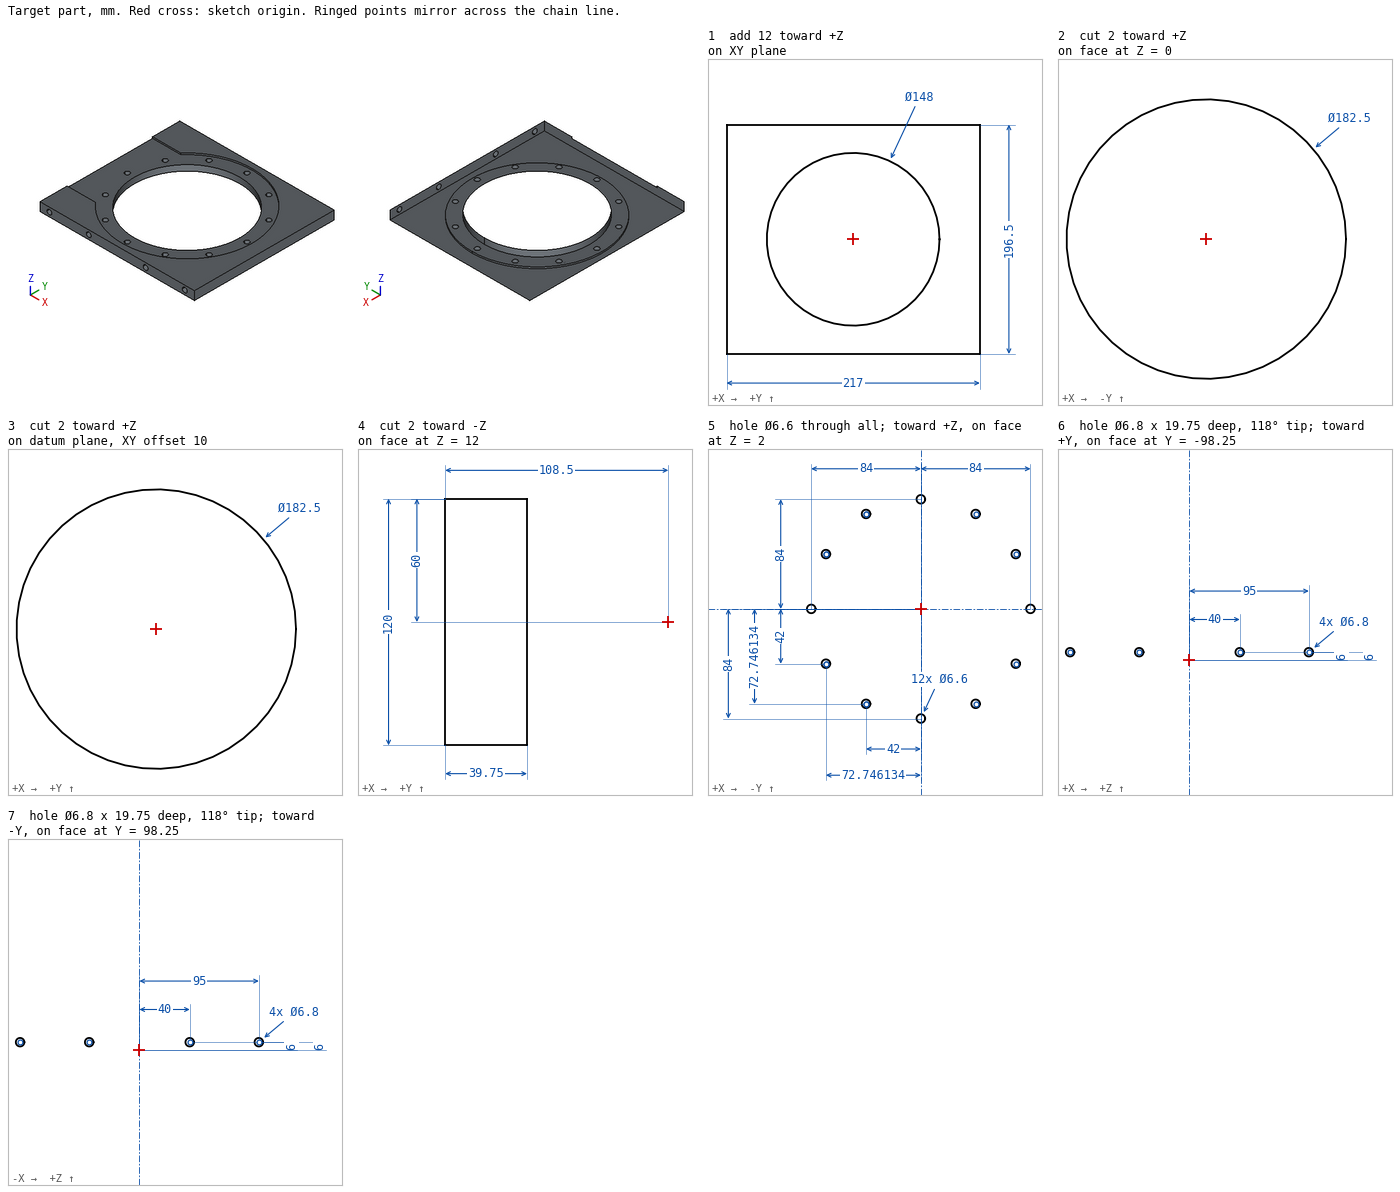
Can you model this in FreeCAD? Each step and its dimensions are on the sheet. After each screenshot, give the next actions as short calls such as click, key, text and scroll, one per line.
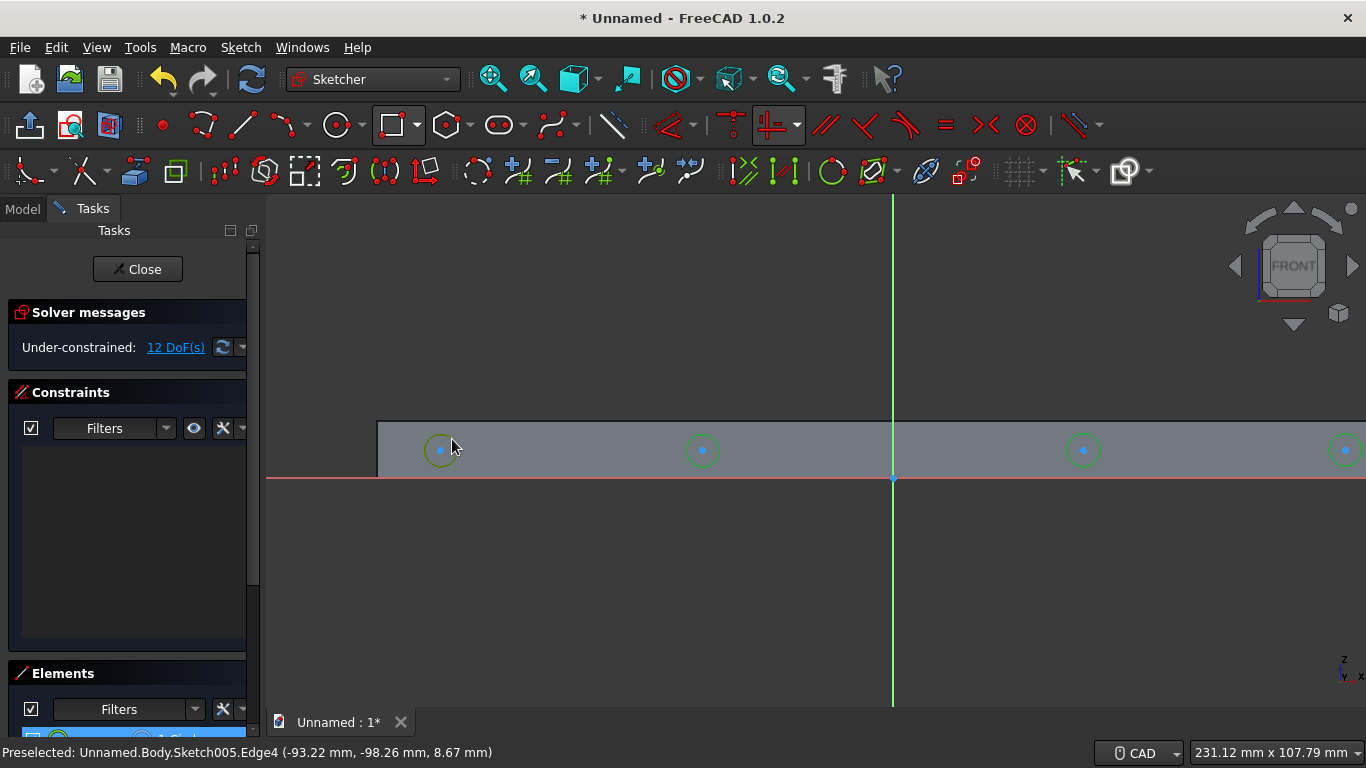
click(946, 126)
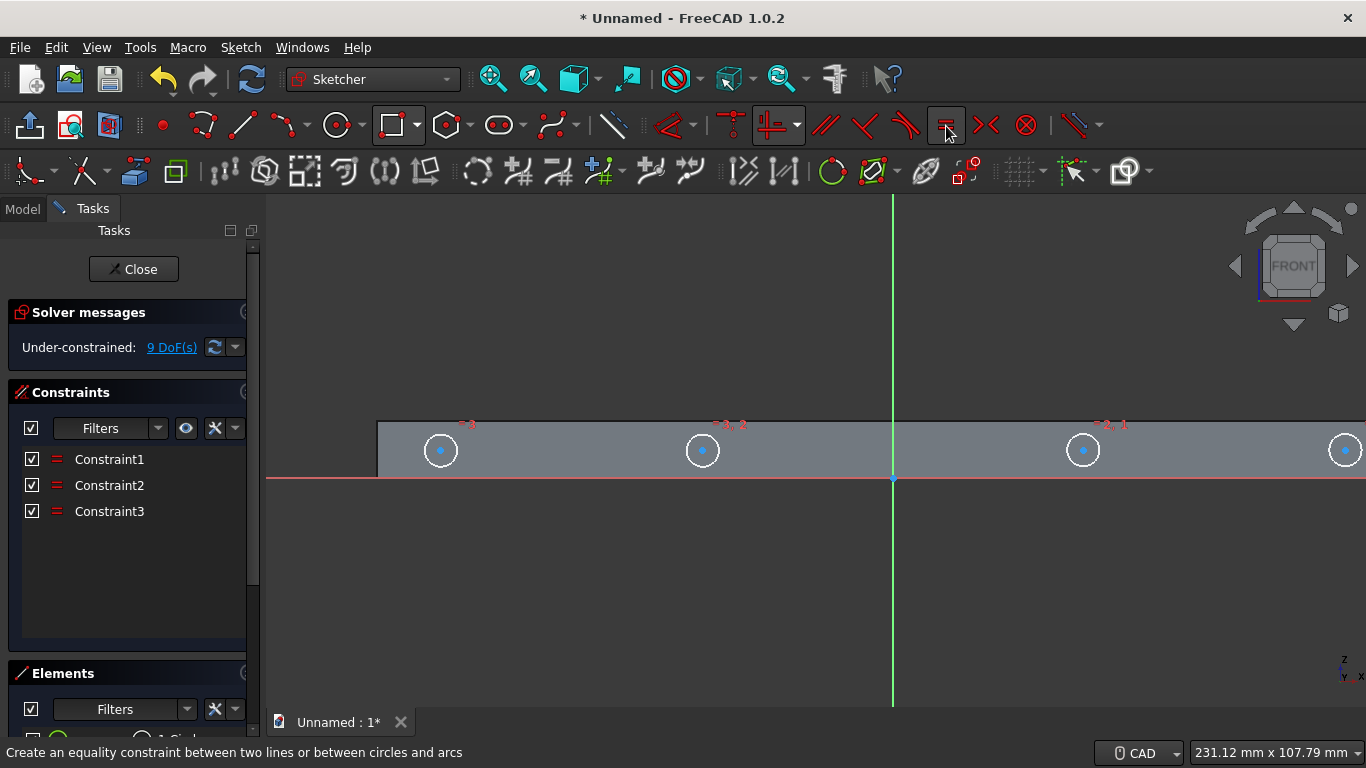
click(1083, 450)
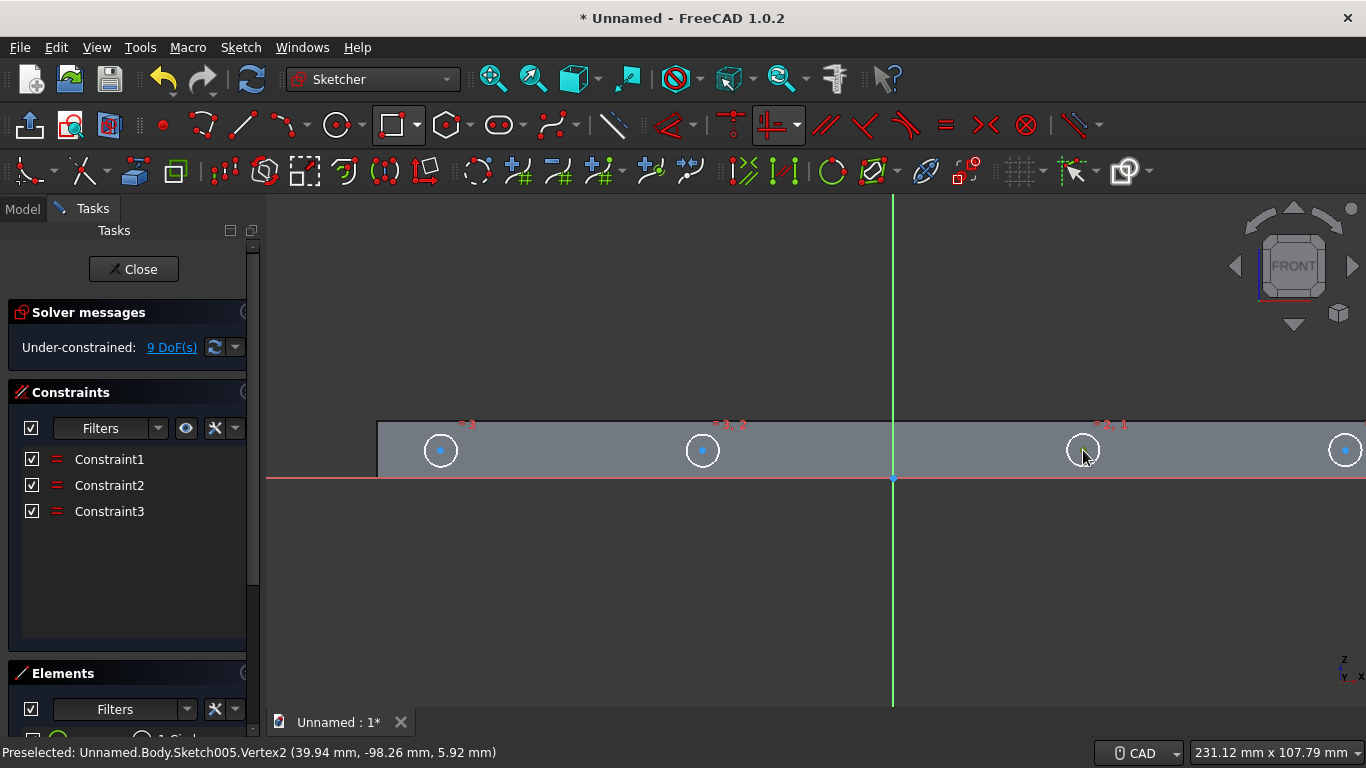
click(703, 451)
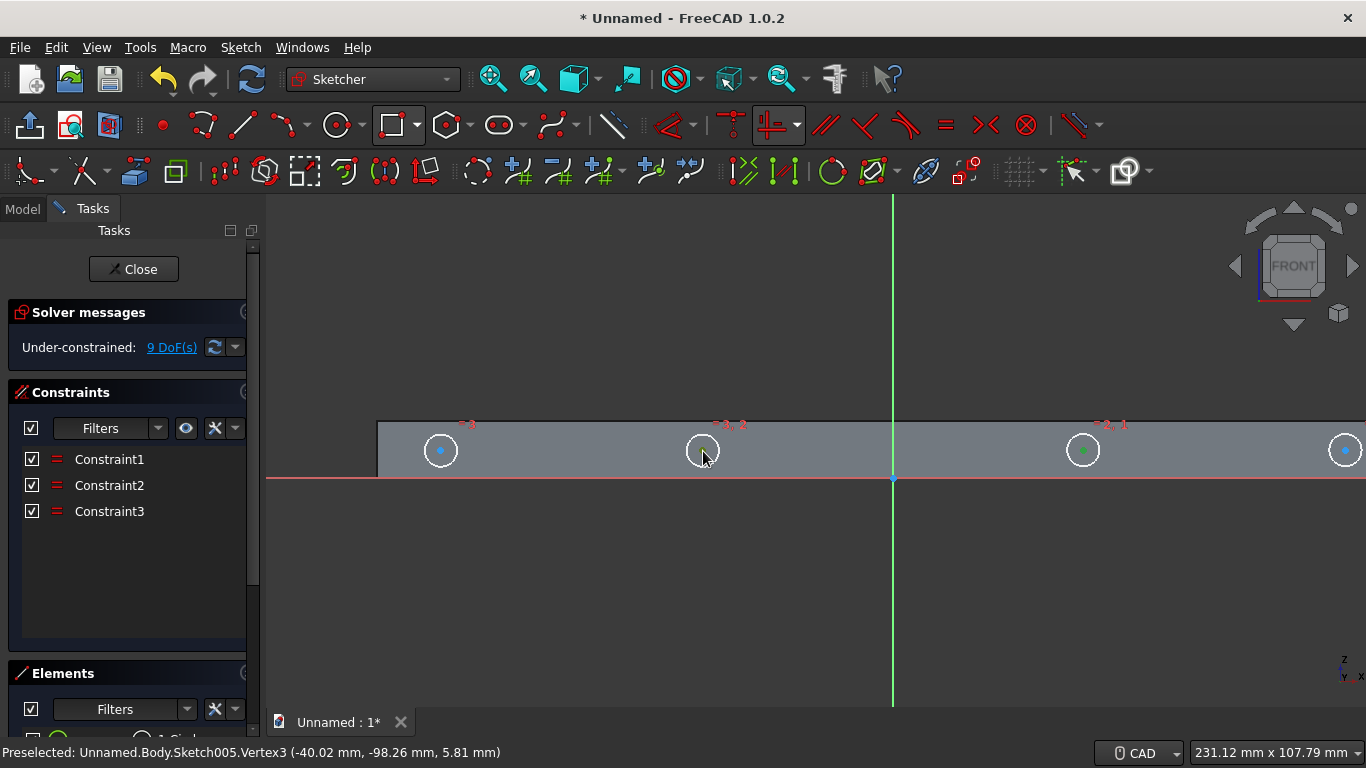
click(893, 646)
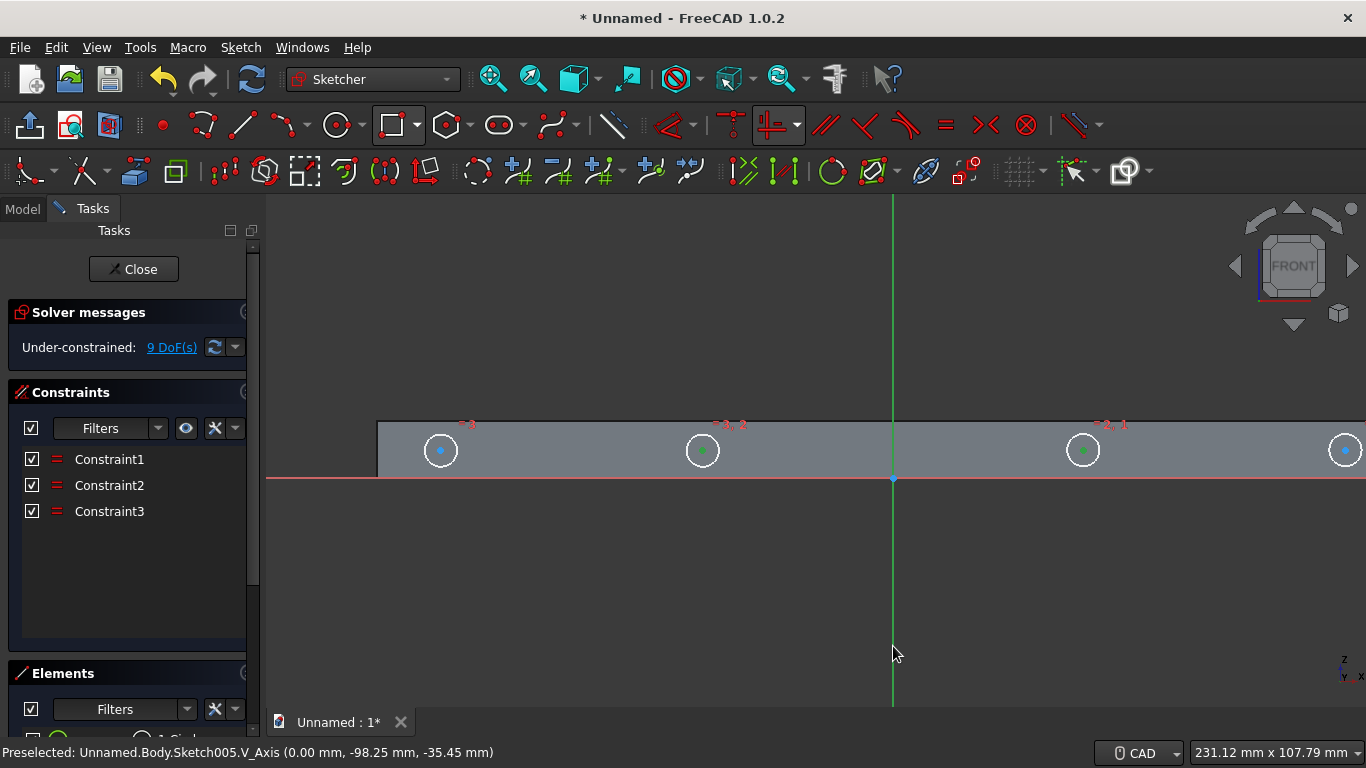
click(986, 126)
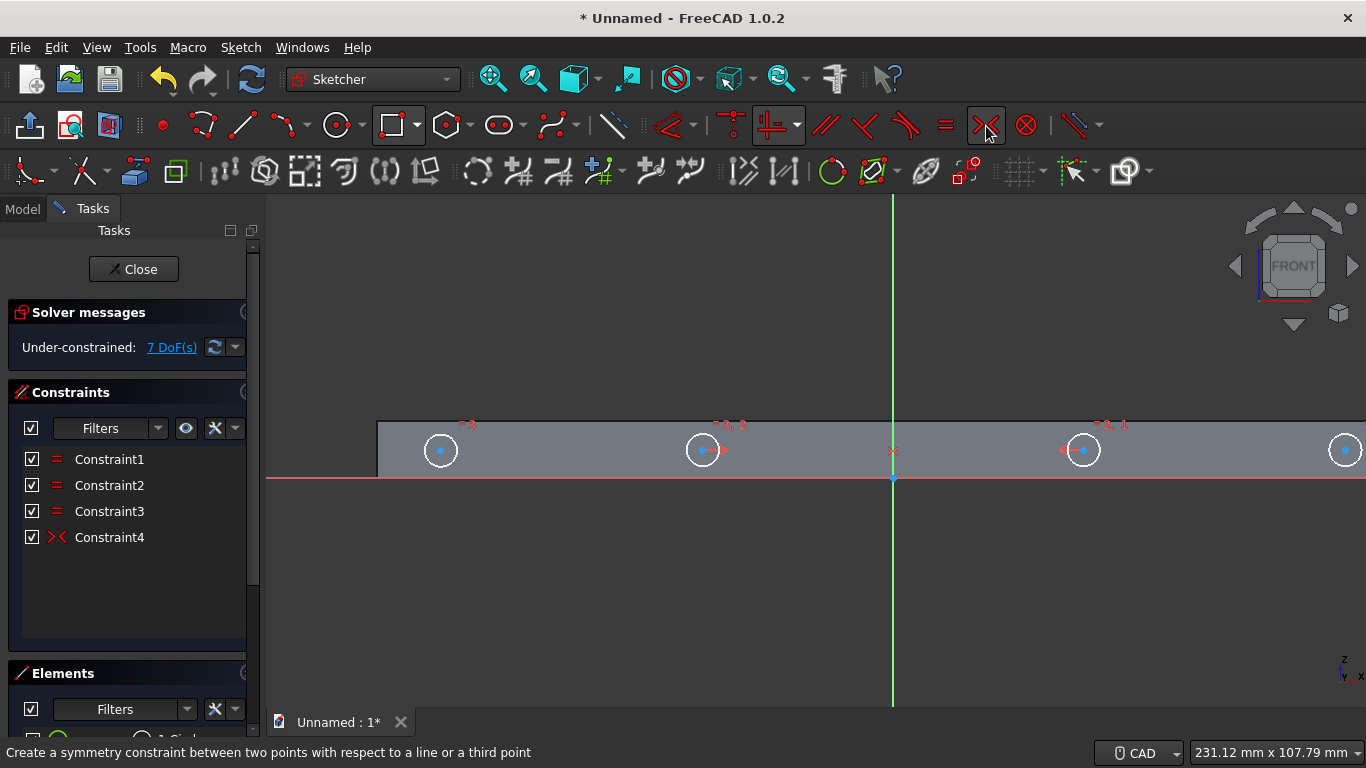
scroll(451, 440, down, 2)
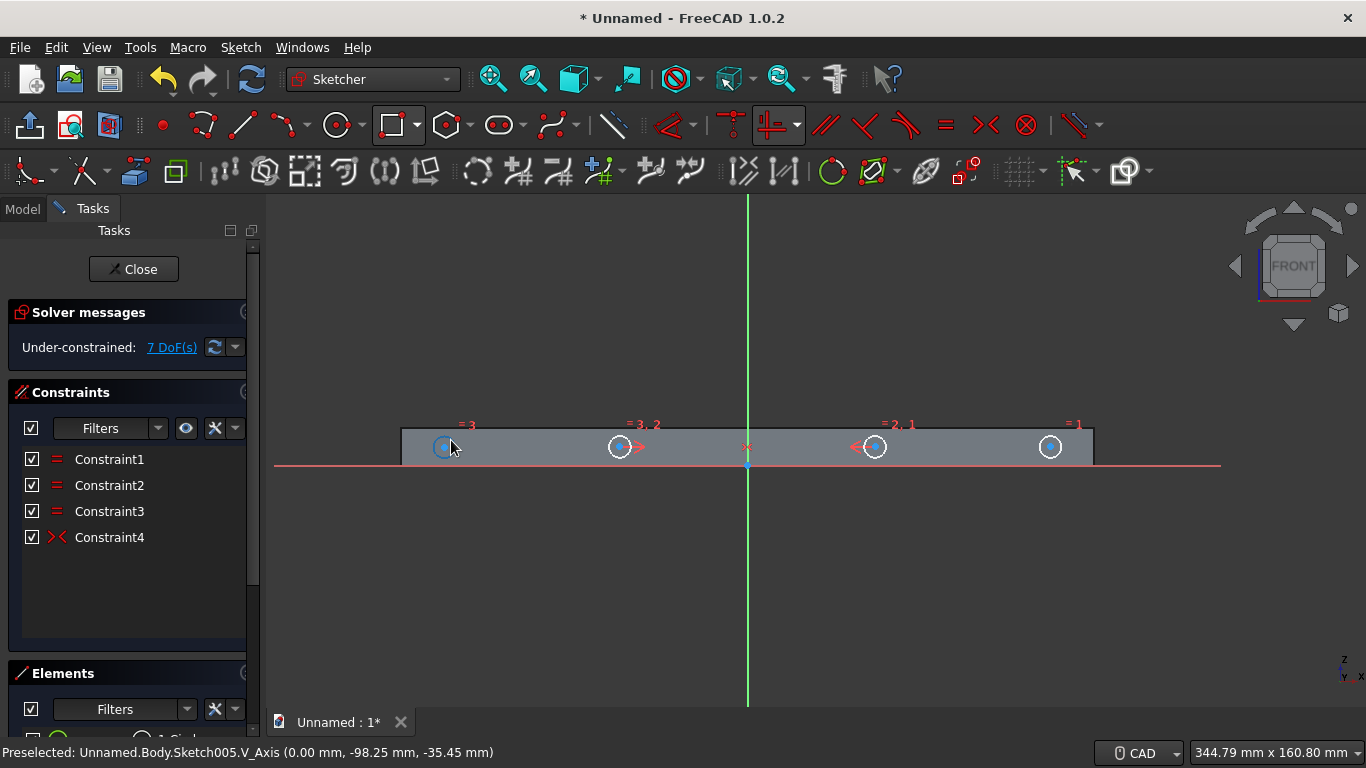
click(1051, 447)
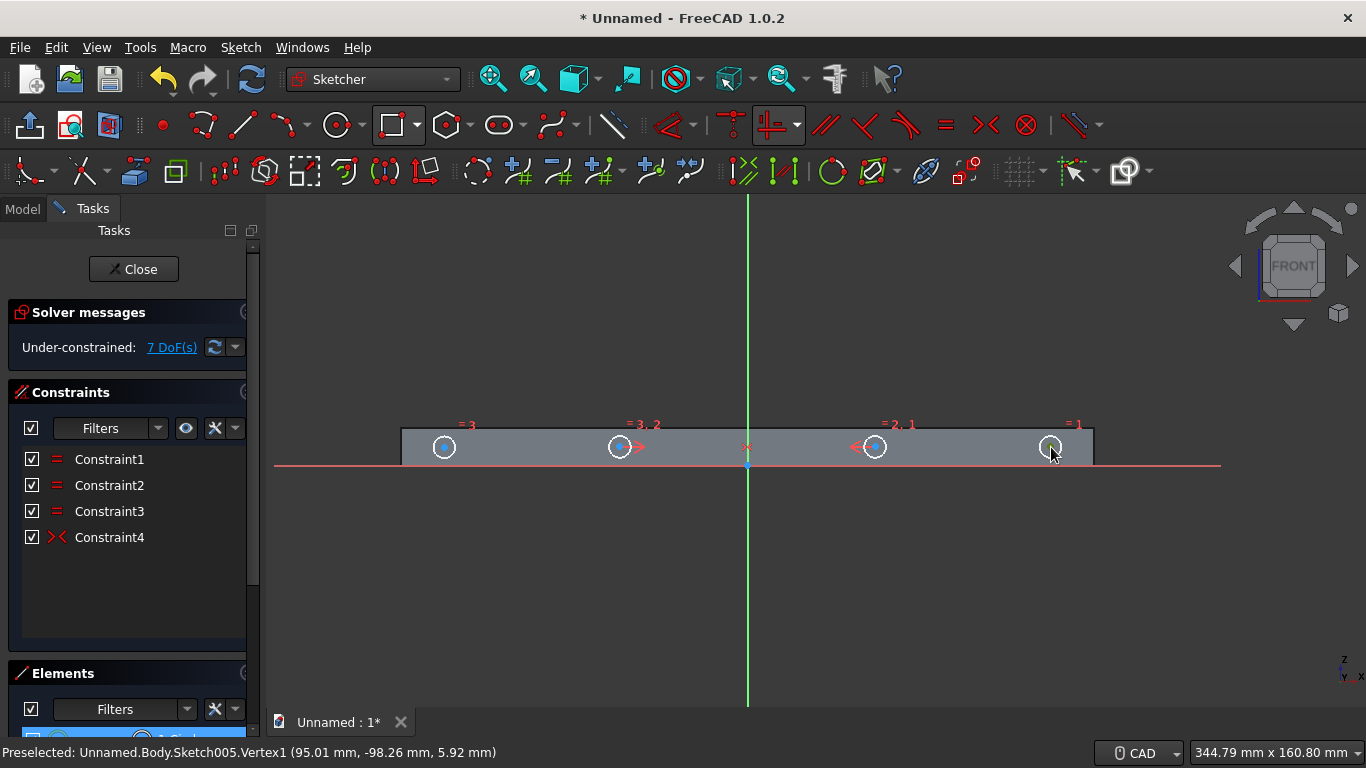
click(444, 447)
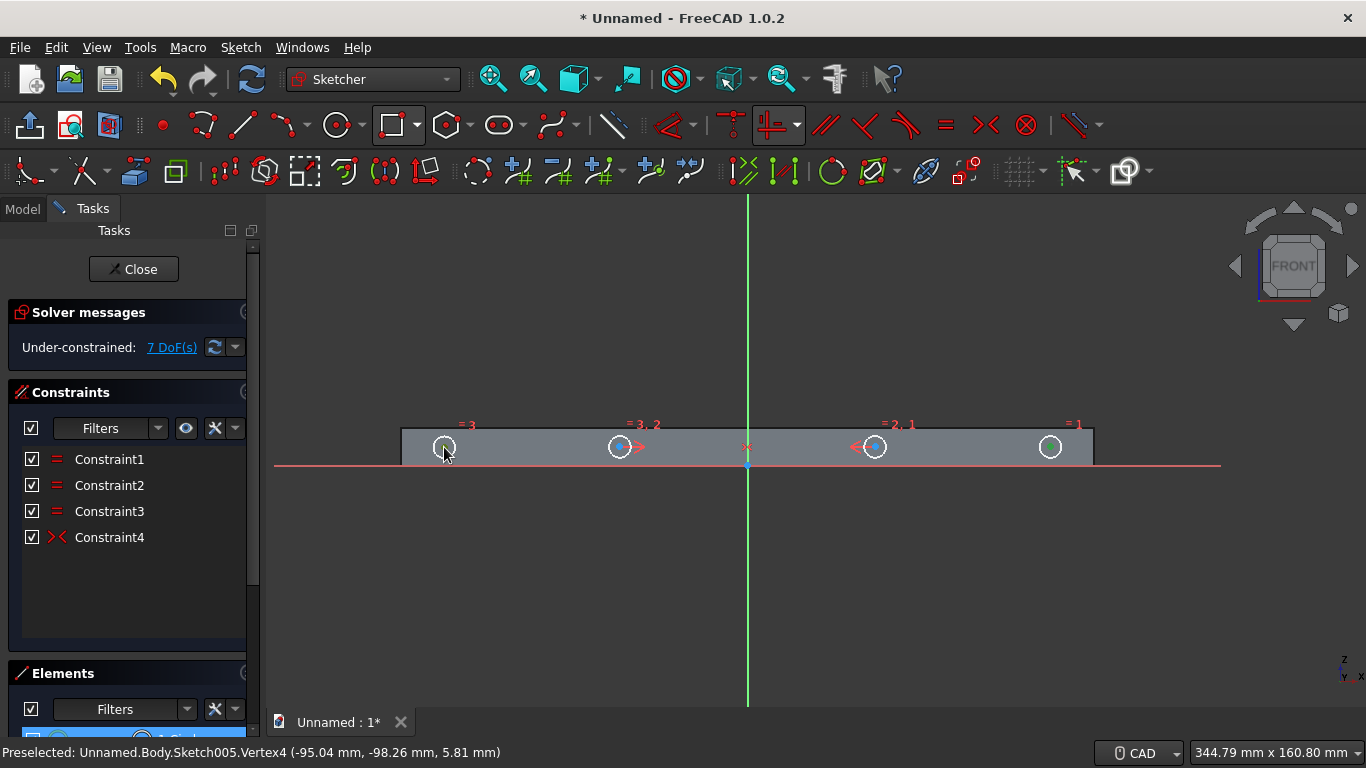
click(748, 646)